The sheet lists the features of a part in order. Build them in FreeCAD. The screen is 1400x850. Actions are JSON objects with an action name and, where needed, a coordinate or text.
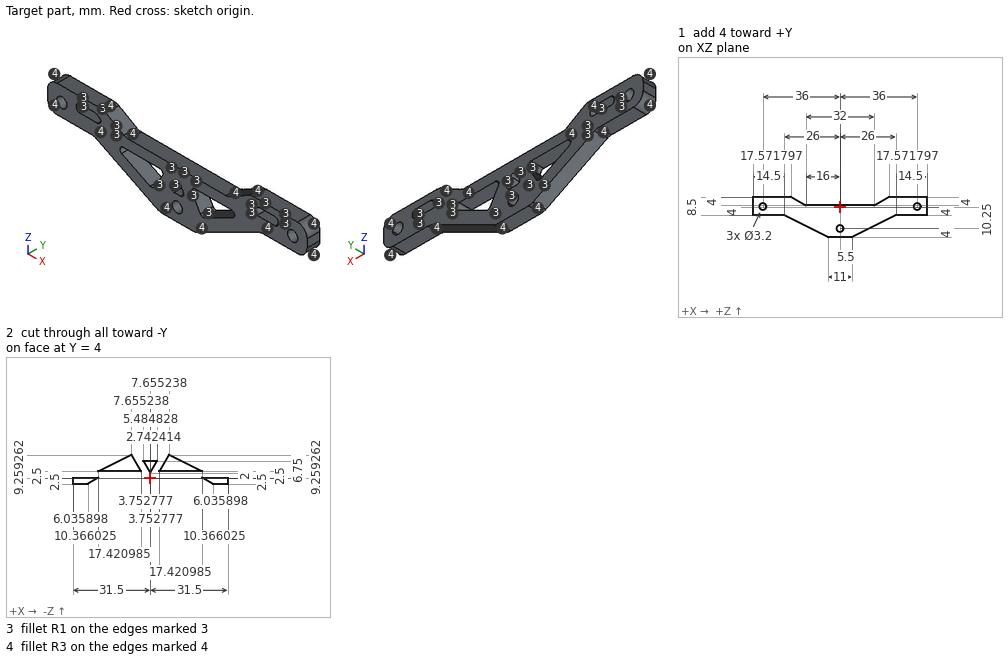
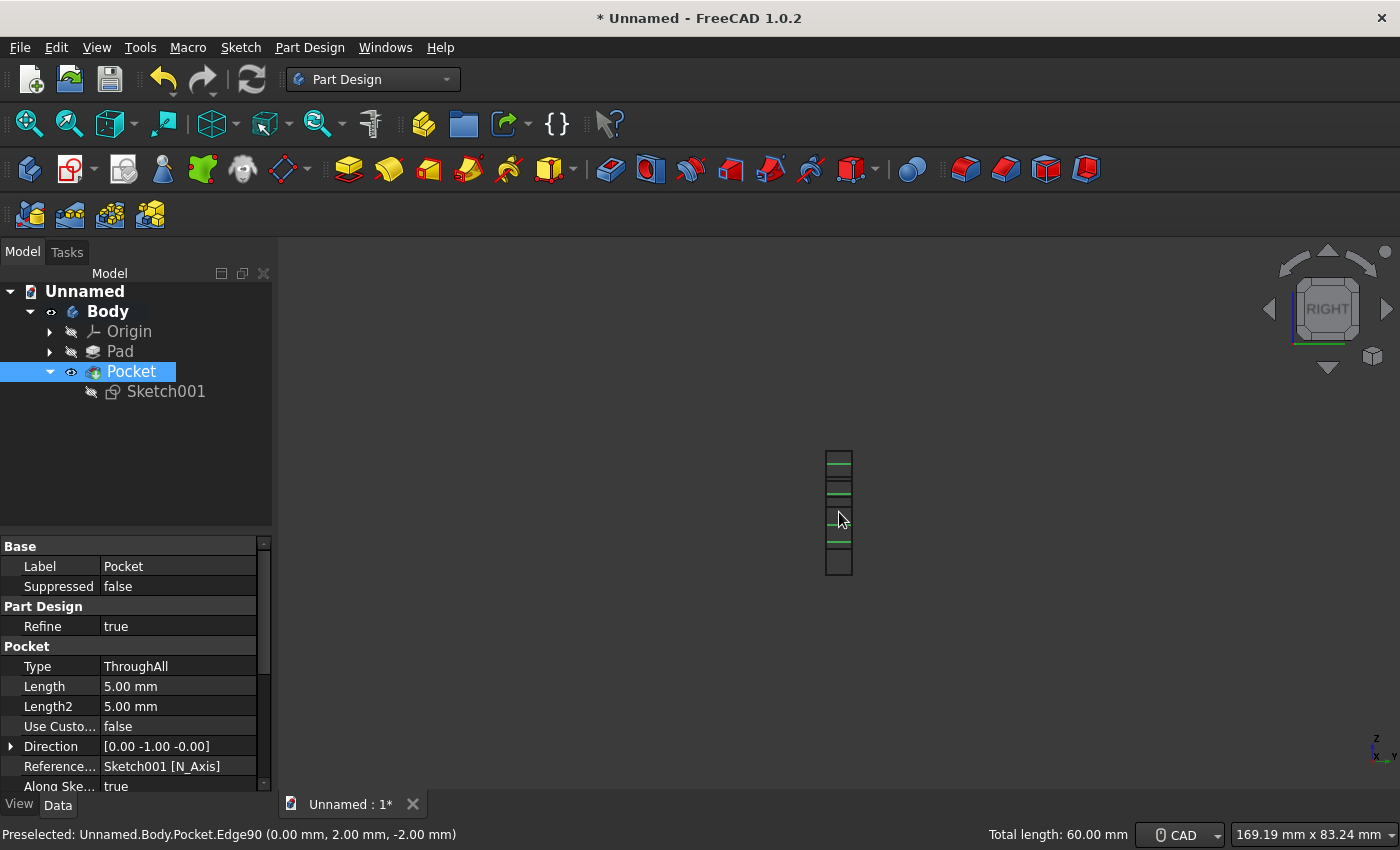
{"action": "left_click", "coordinate": [30, 124]}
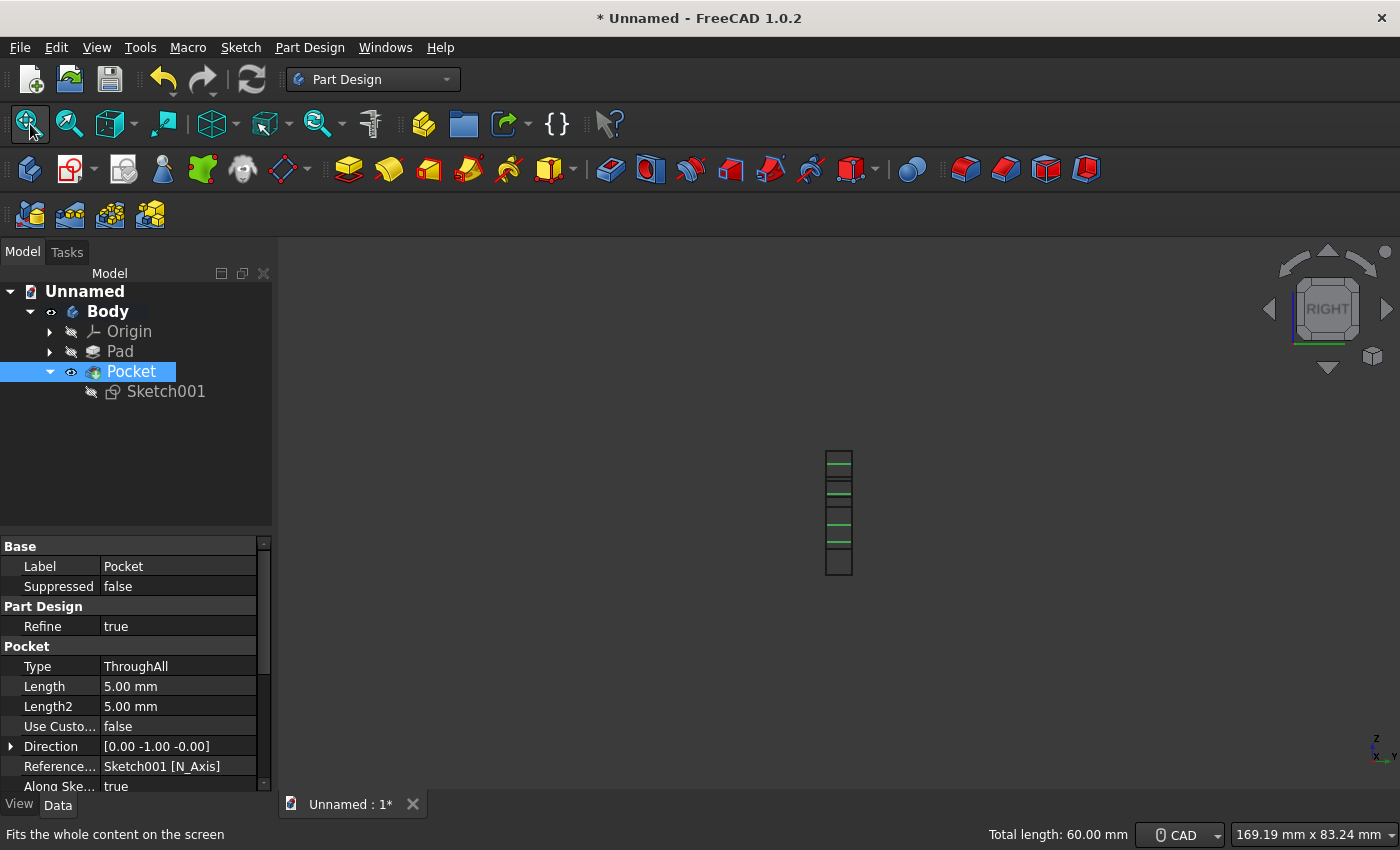
{"action": "left_click", "coordinate": [839, 496], "text": "ctrl"}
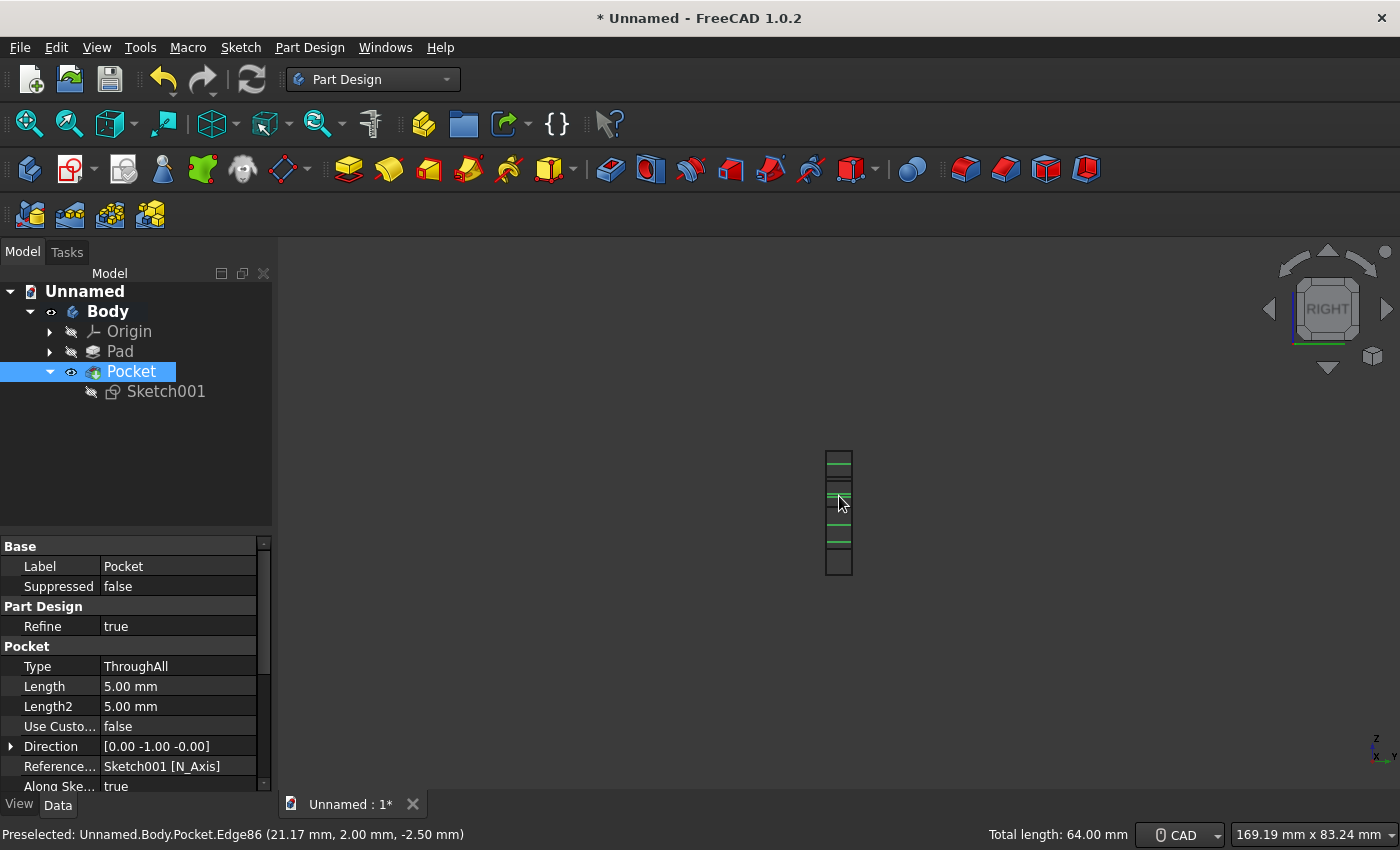
{"action": "key", "text": "5"}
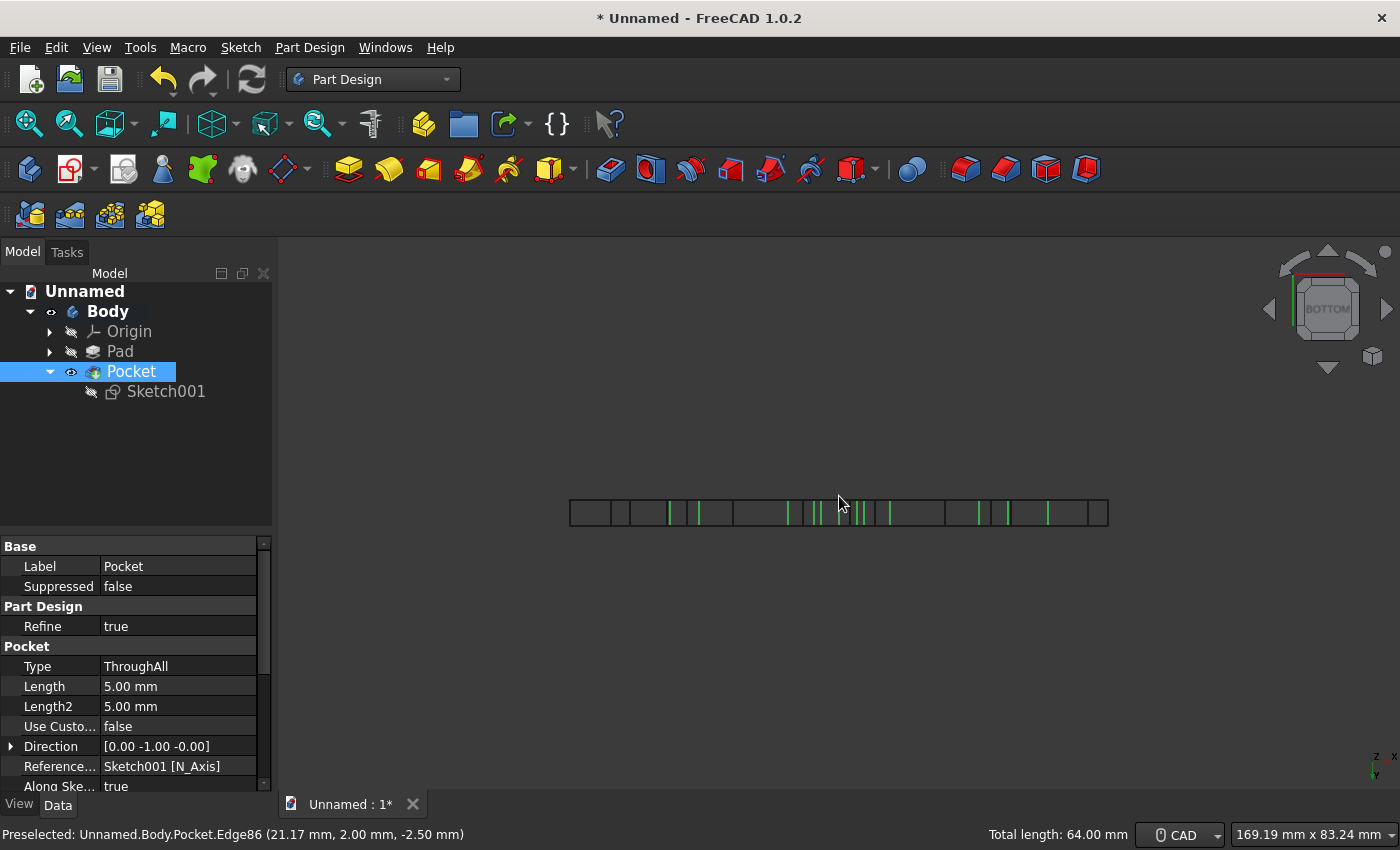
{"action": "left_click", "coordinate": [630, 512], "text": "ctrl"}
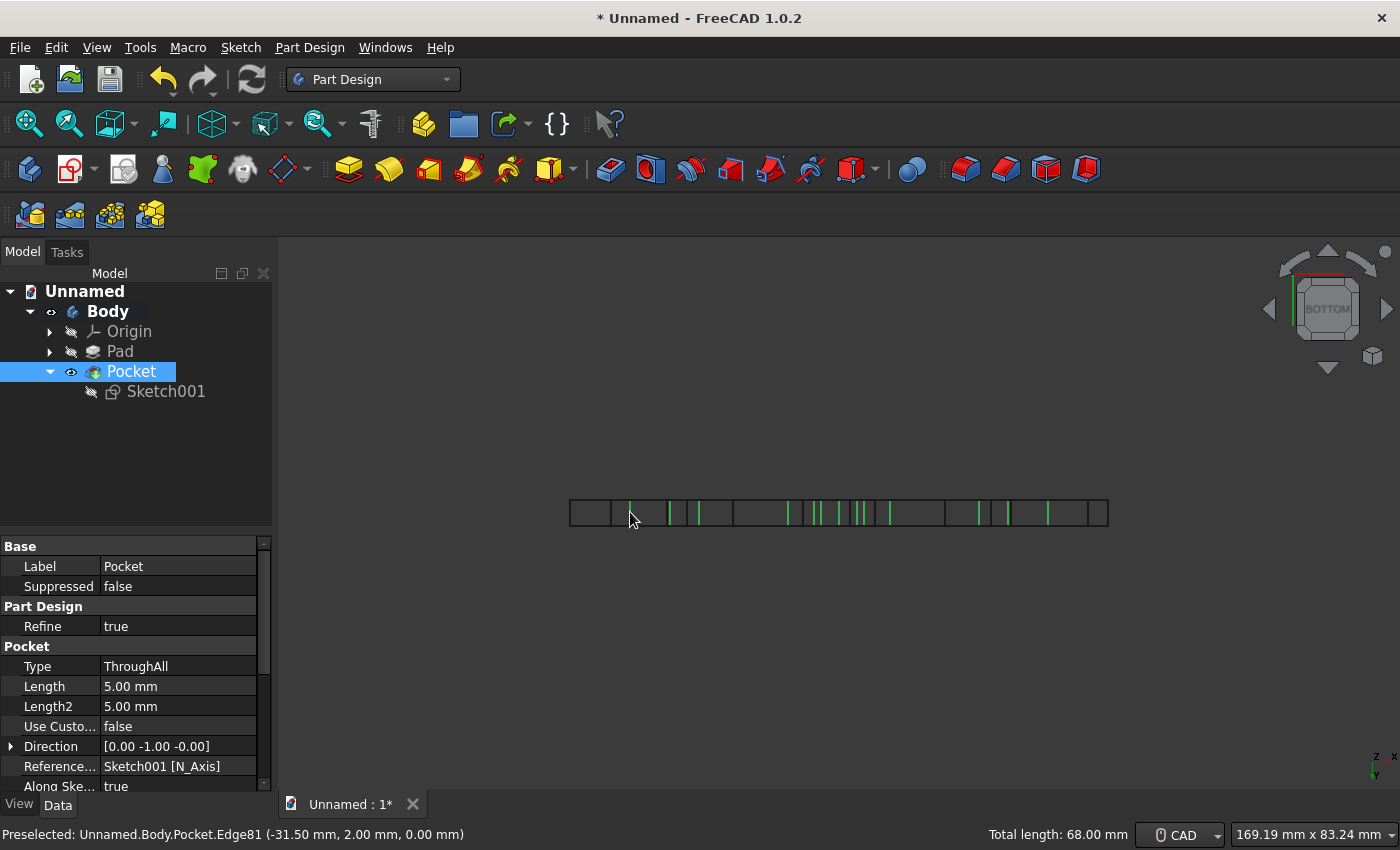
{"action": "key", "text": "v 1"}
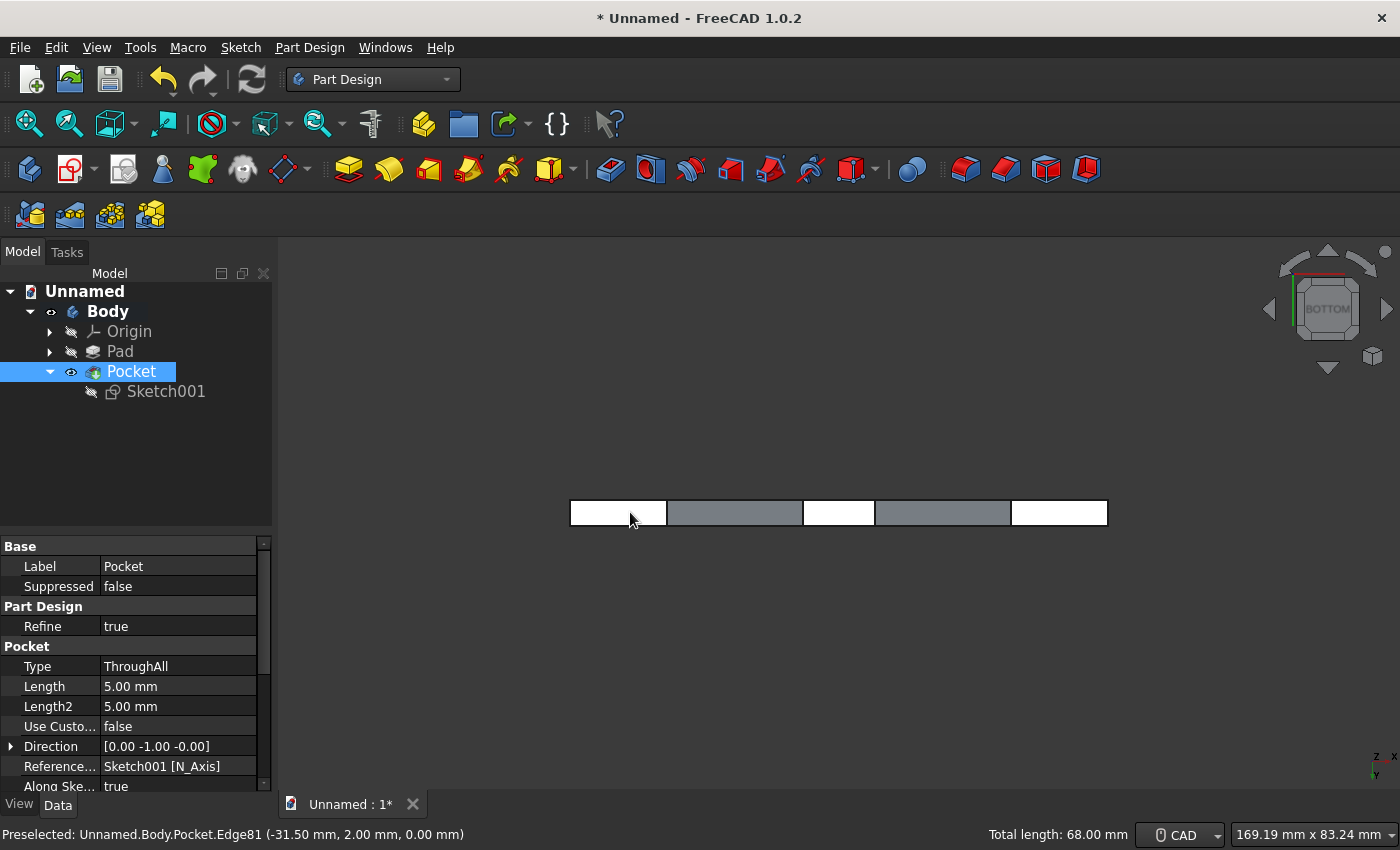
{"action": "left_click", "coordinate": [966, 170]}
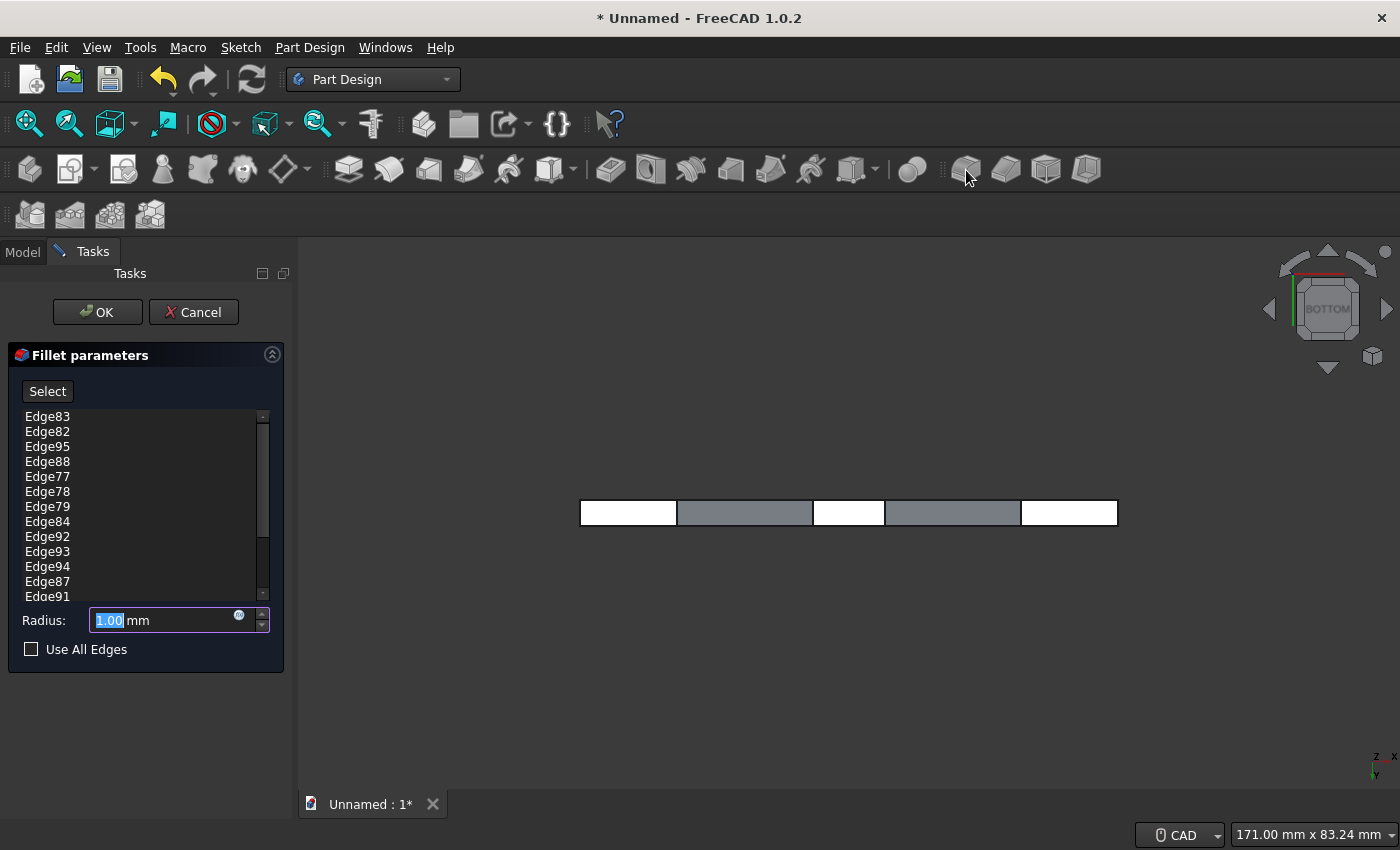
{"action": "type", "text": "1"}
{"action": "key", "text": "Tab"}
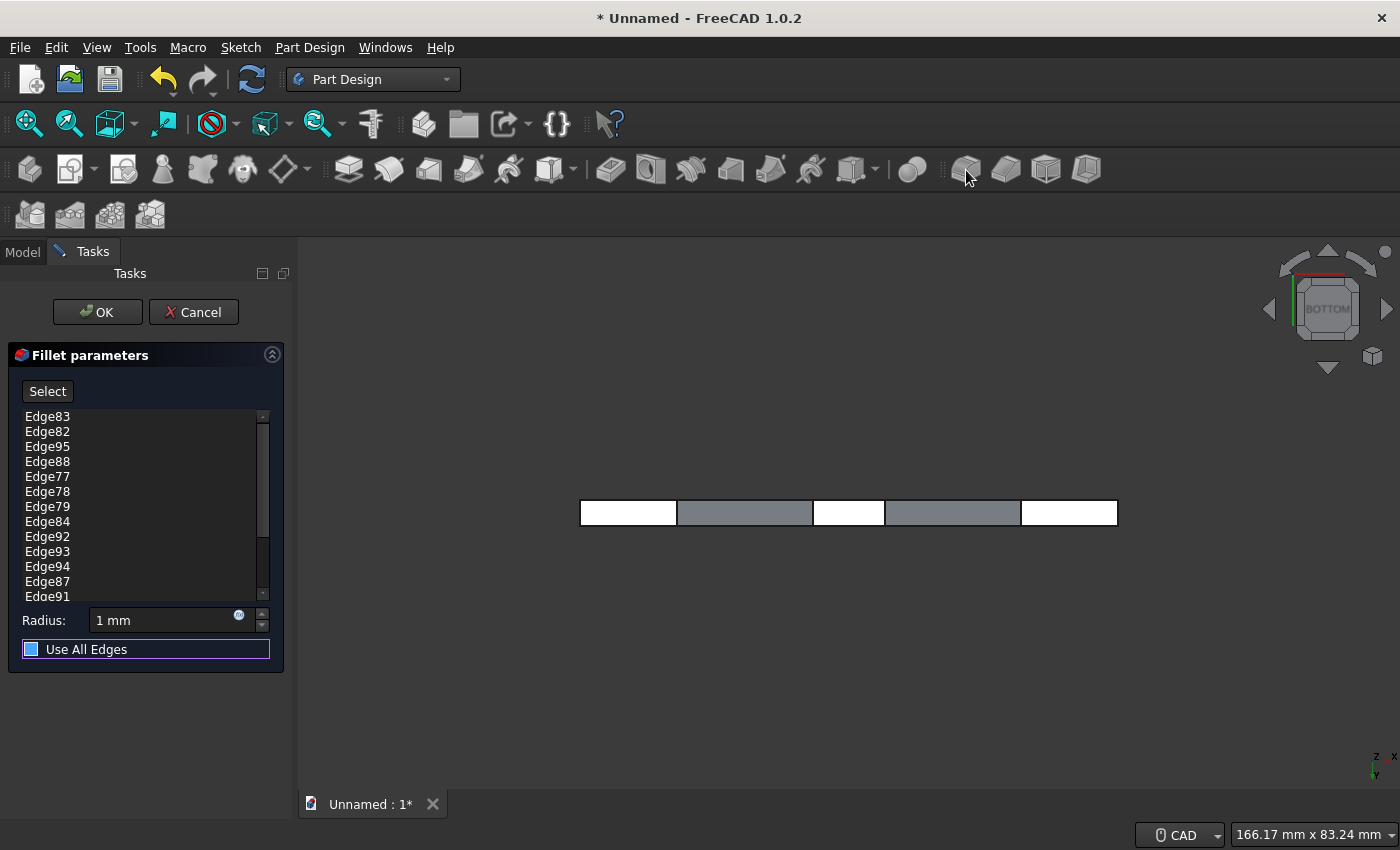
{"action": "left_click", "coordinate": [98, 312]}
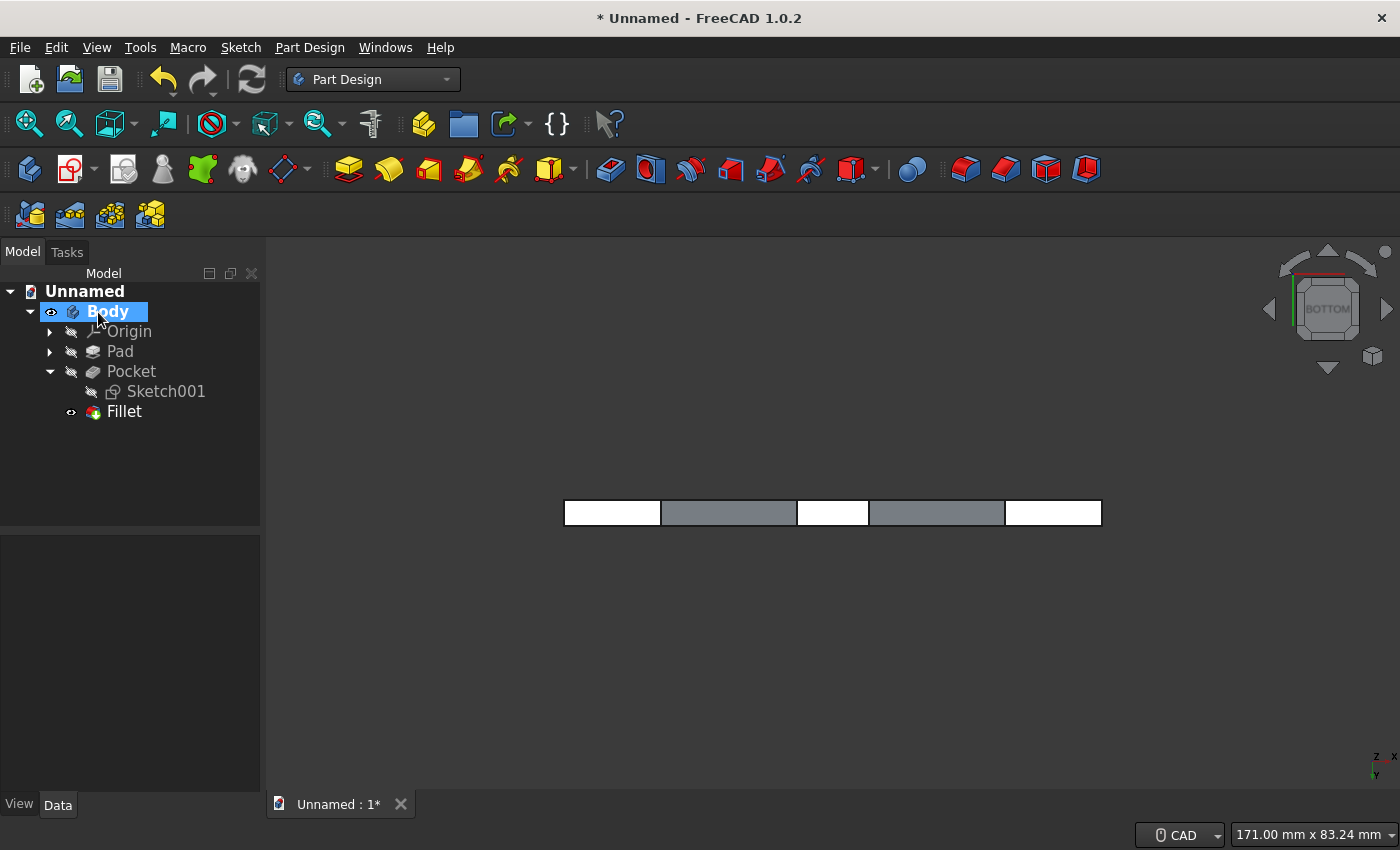
{"action": "left_click", "coordinate": [1102, 512]}